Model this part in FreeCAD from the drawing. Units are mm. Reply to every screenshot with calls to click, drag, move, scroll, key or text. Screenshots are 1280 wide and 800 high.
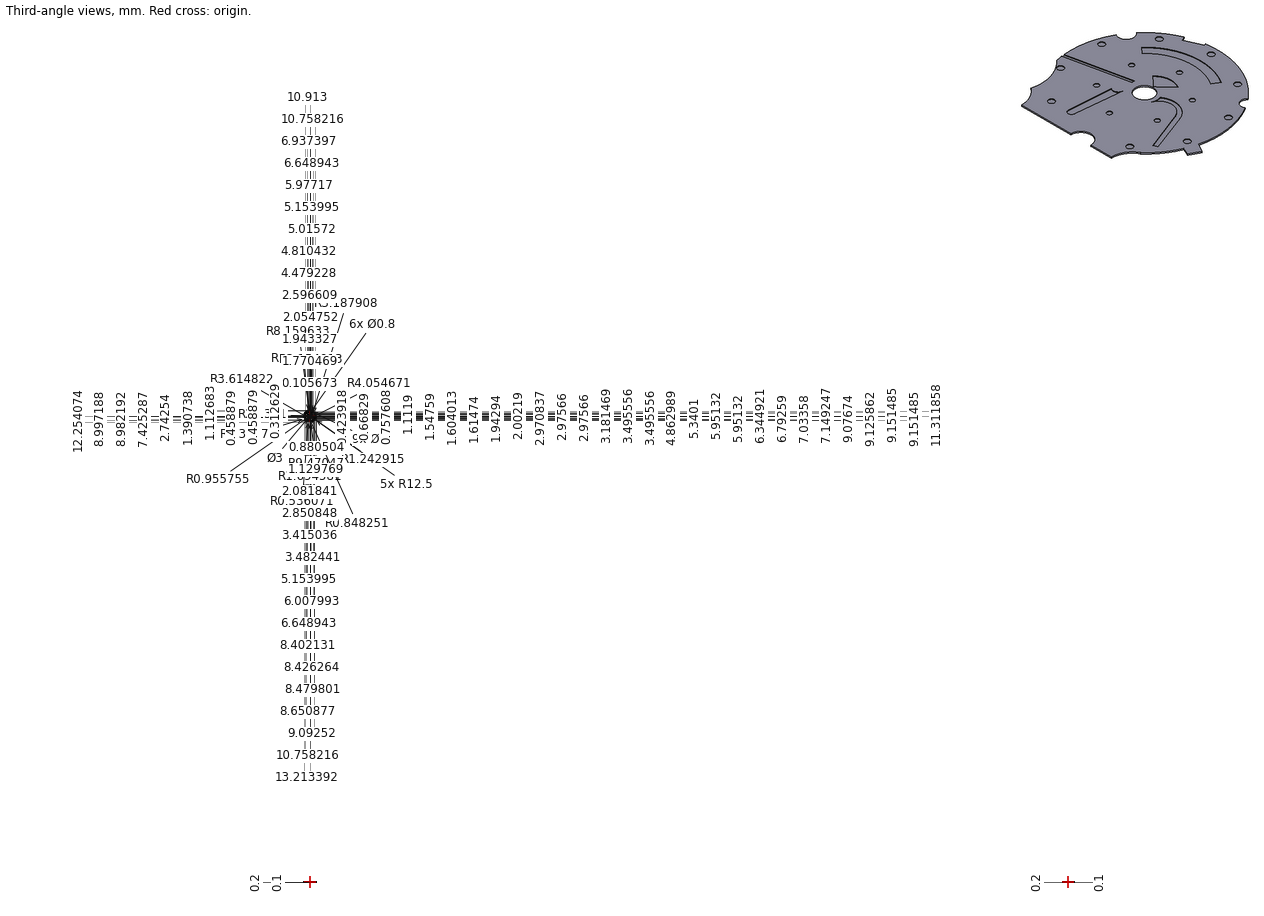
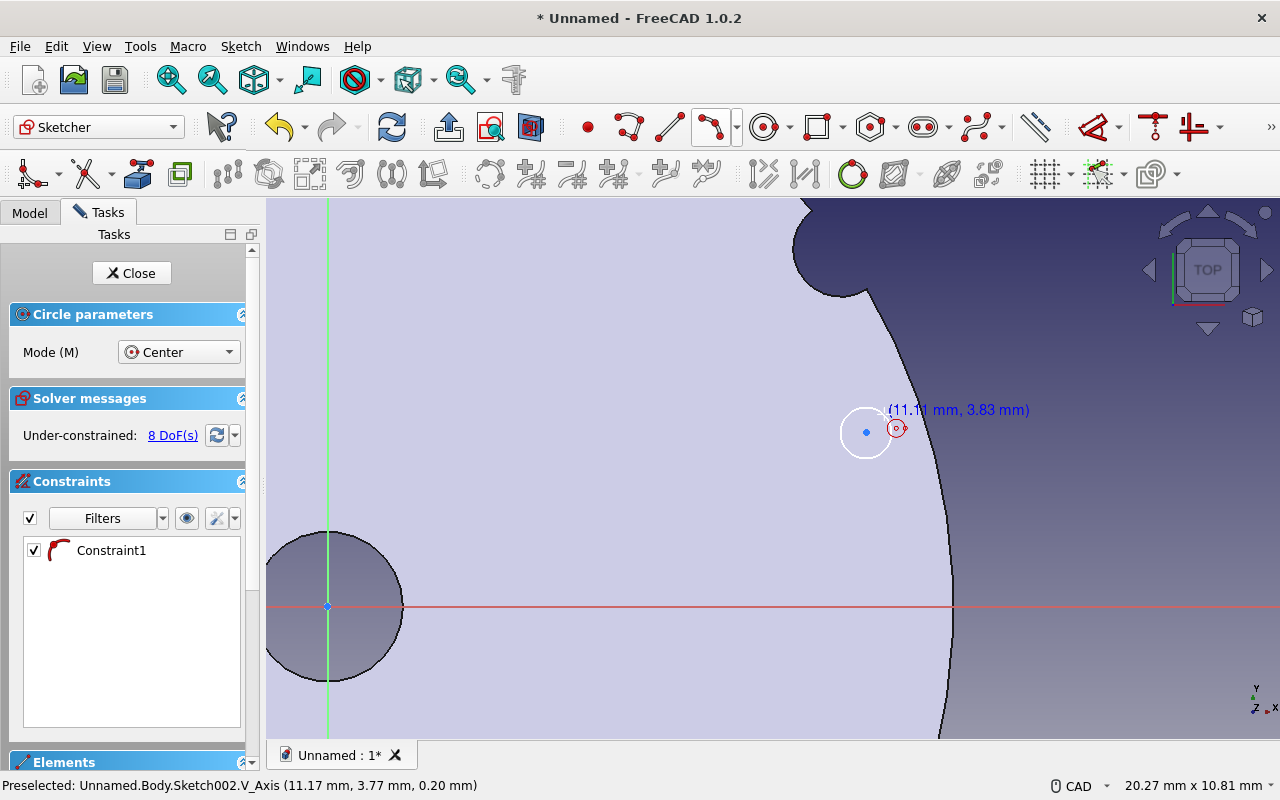
scroll(867, 432, down, 6)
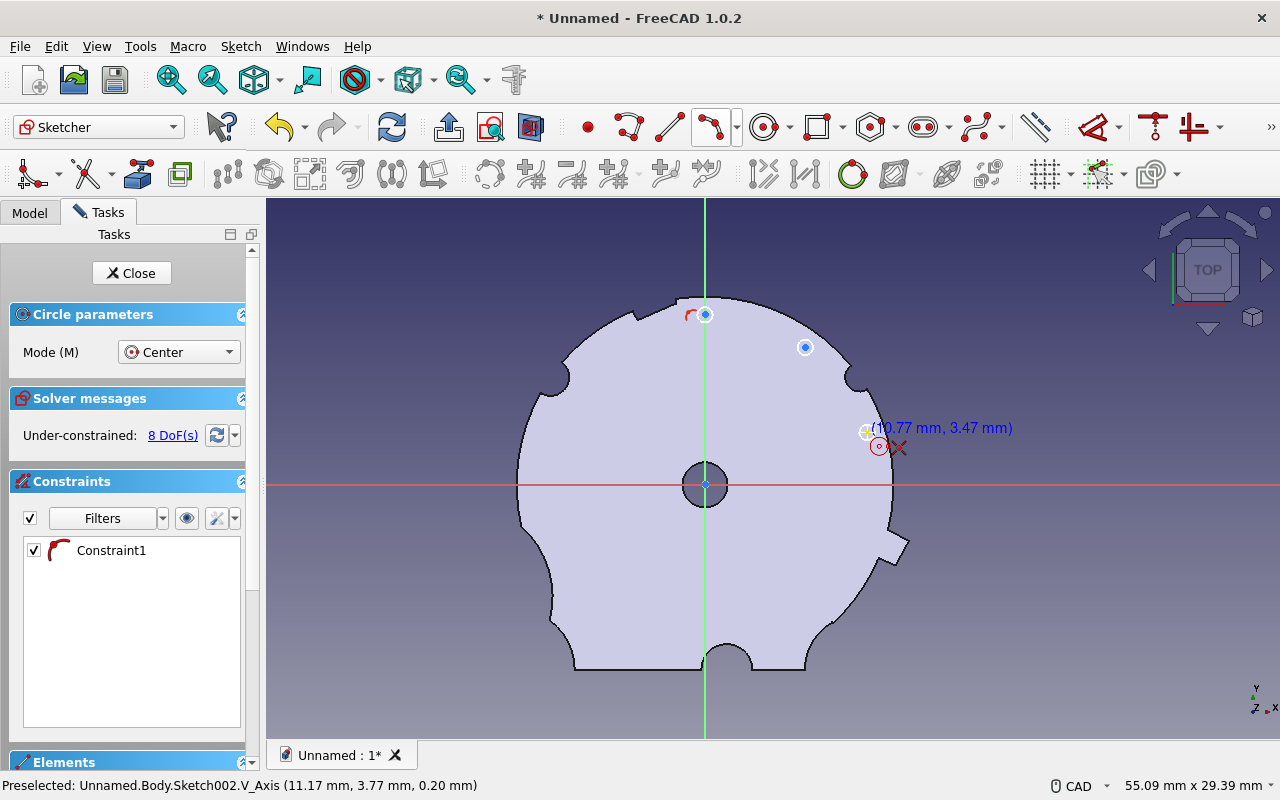
scroll(867, 538, up, 6)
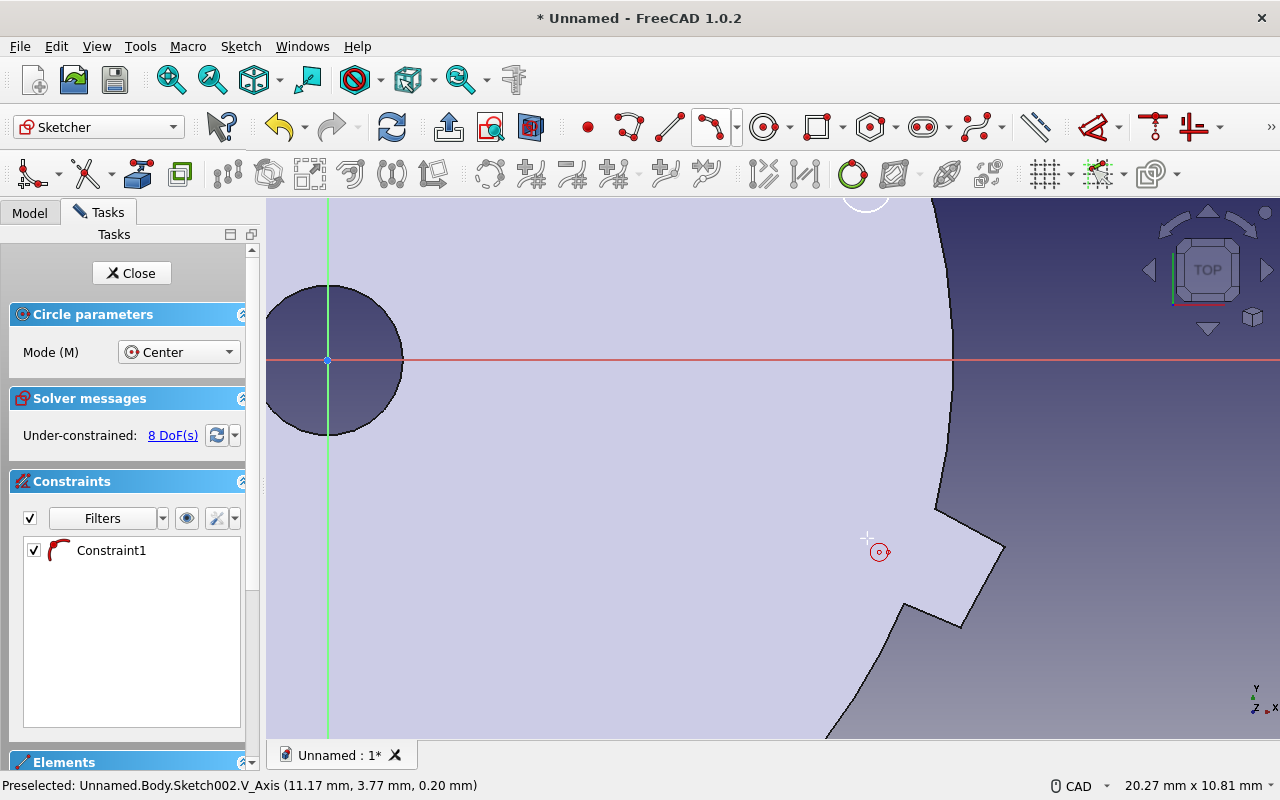
click(866, 535)
click(884, 518)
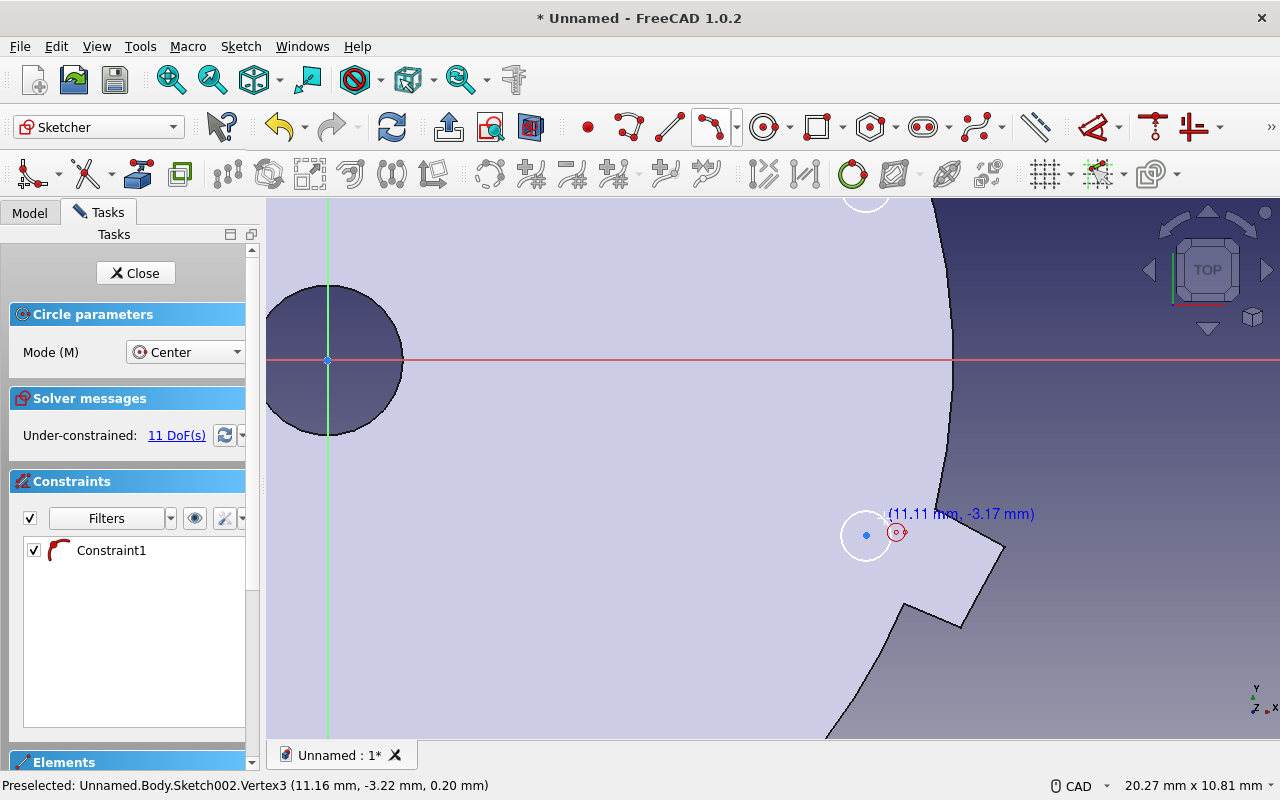
scroll(867, 538, down, 6)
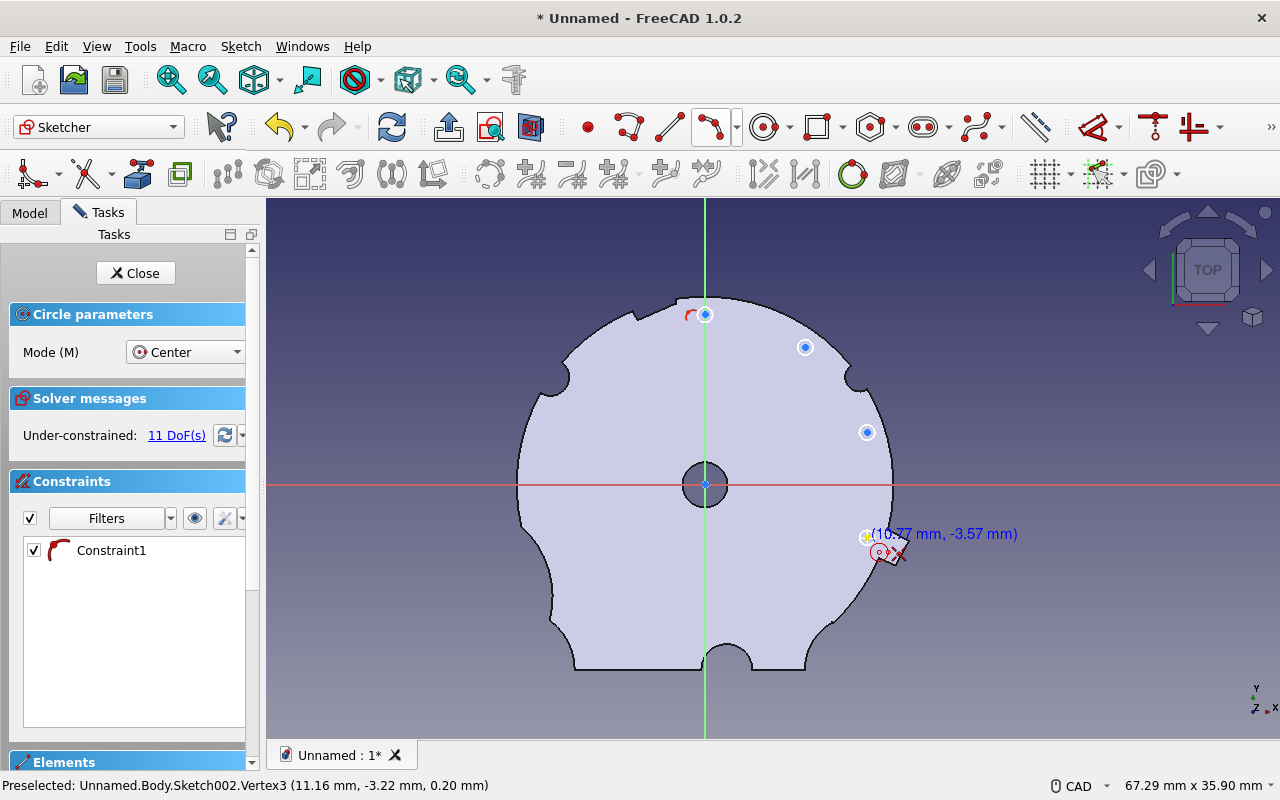
scroll(805, 623, up, 6)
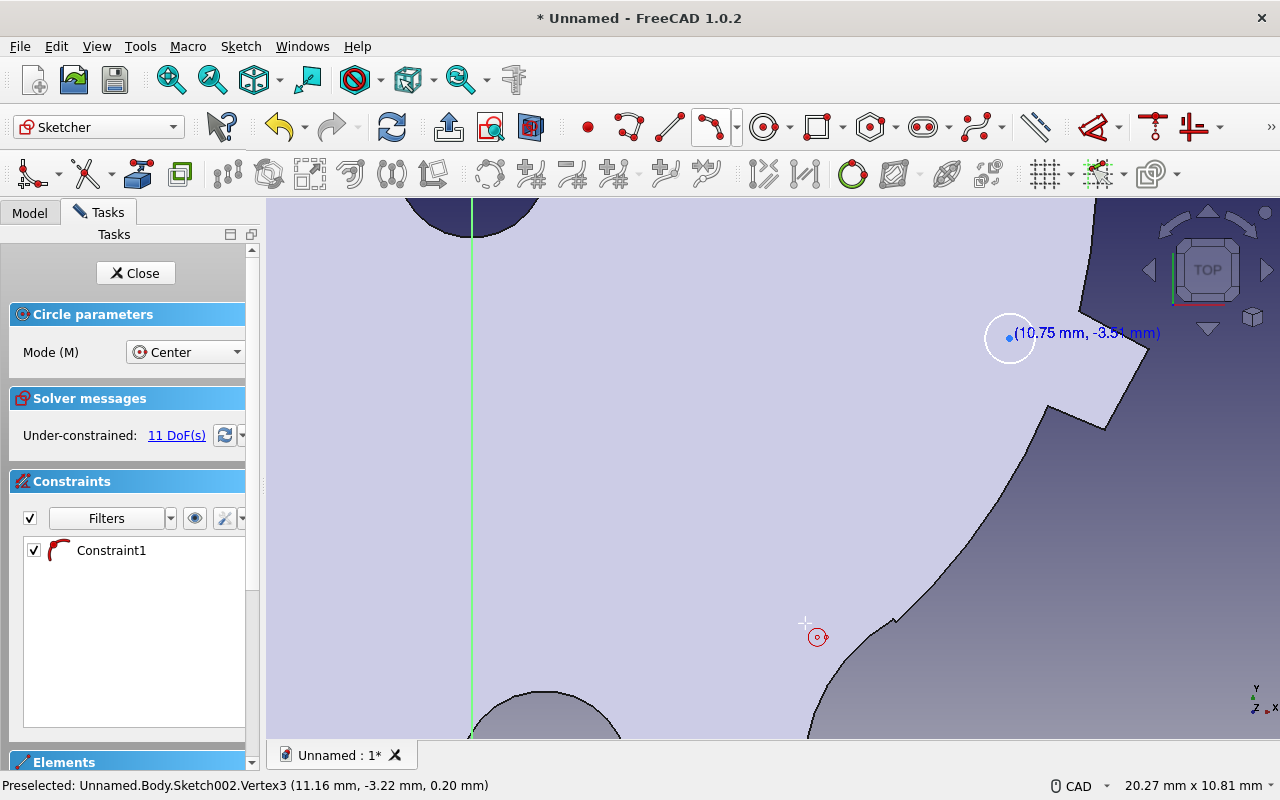
click(805, 621)
click(822, 603)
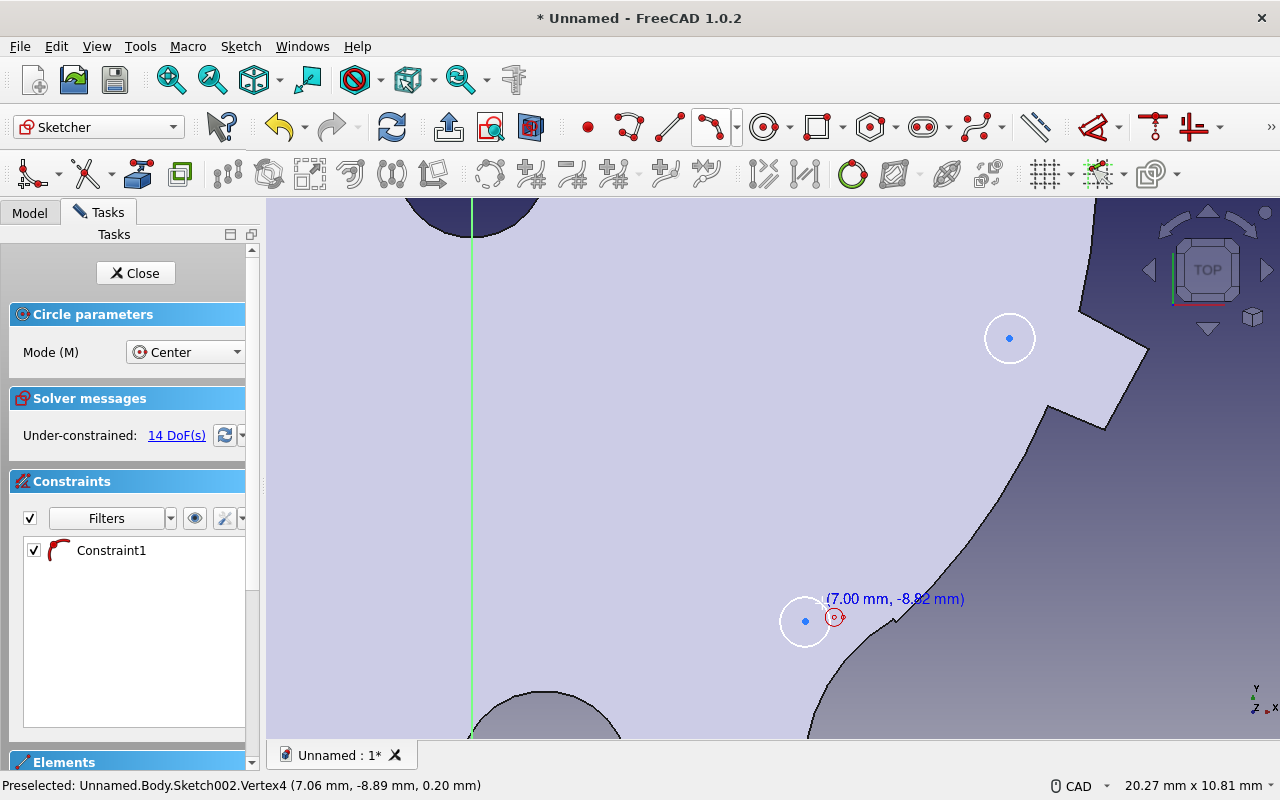
scroll(805, 624, down, 6)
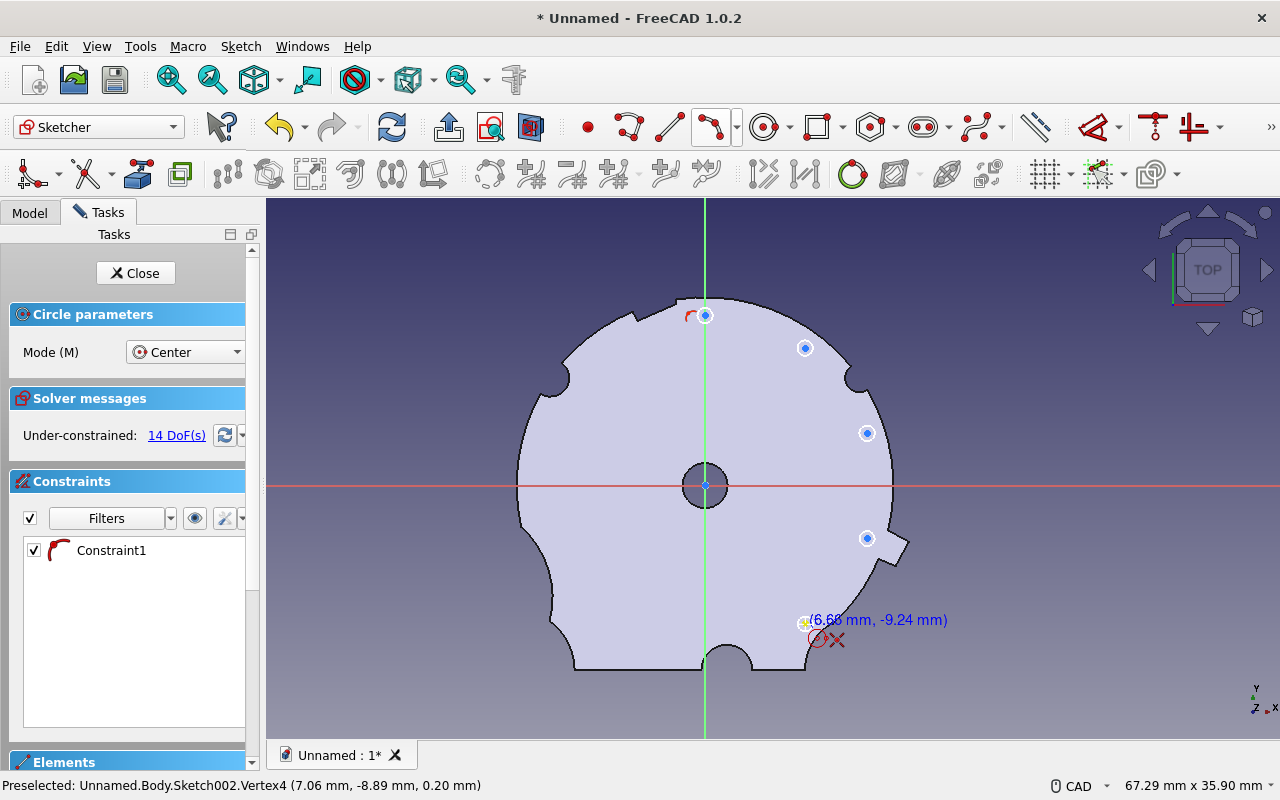
scroll(605, 624, up, 6)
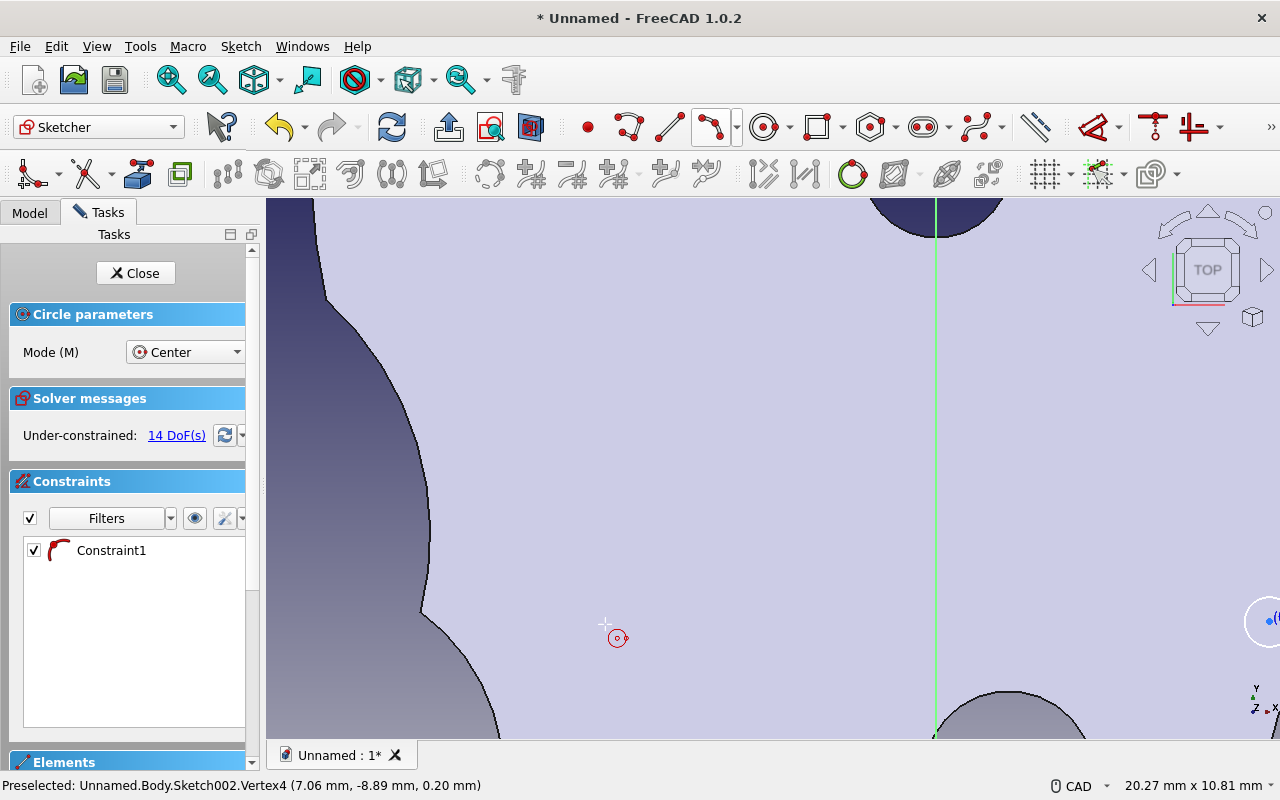
click(604, 621)
click(621, 603)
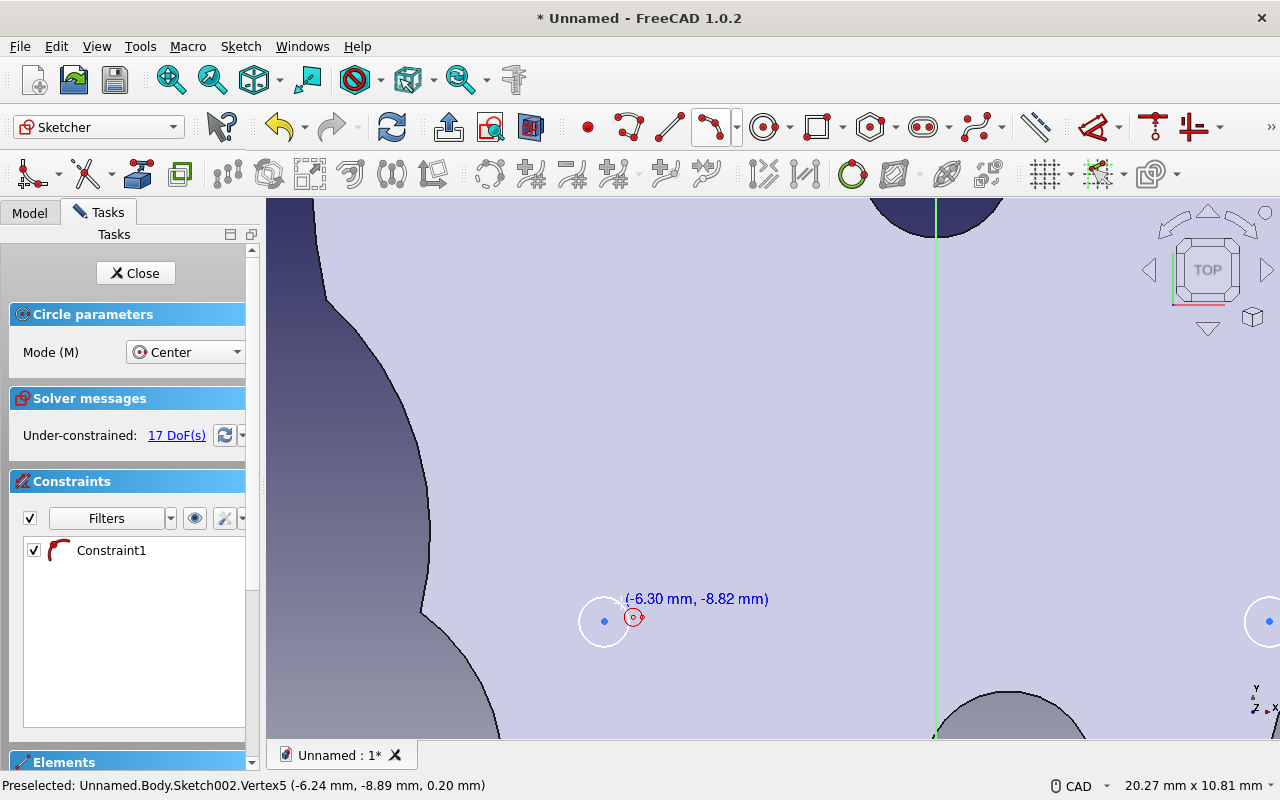
click(398, 338)
click(416, 320)